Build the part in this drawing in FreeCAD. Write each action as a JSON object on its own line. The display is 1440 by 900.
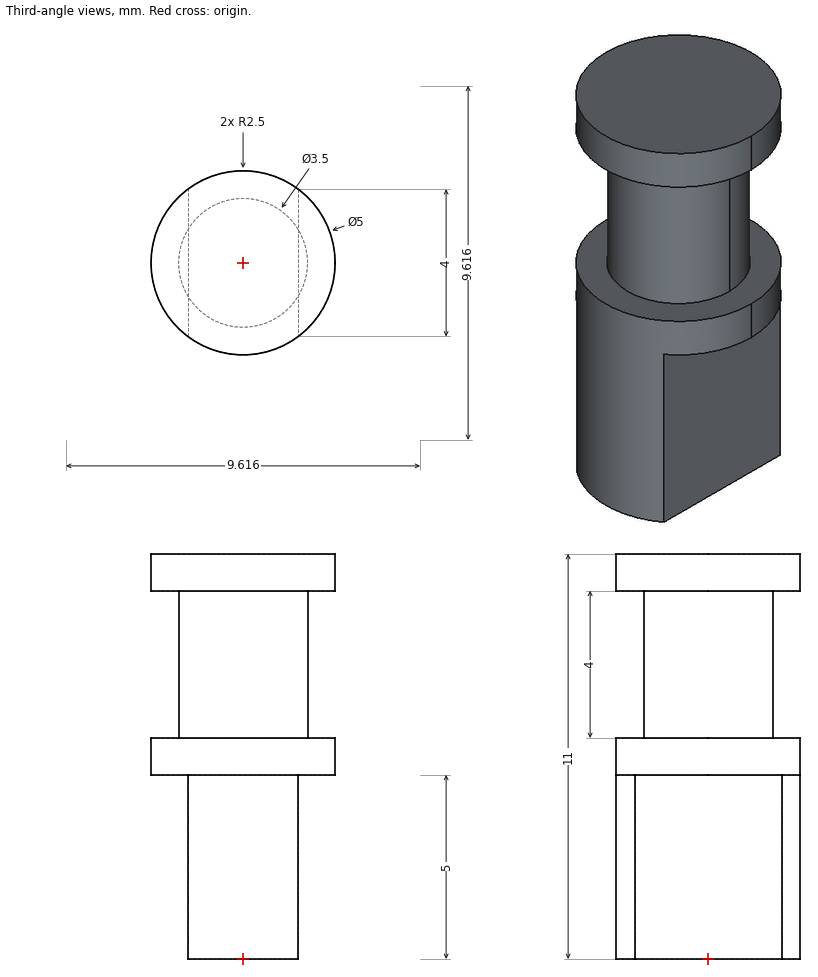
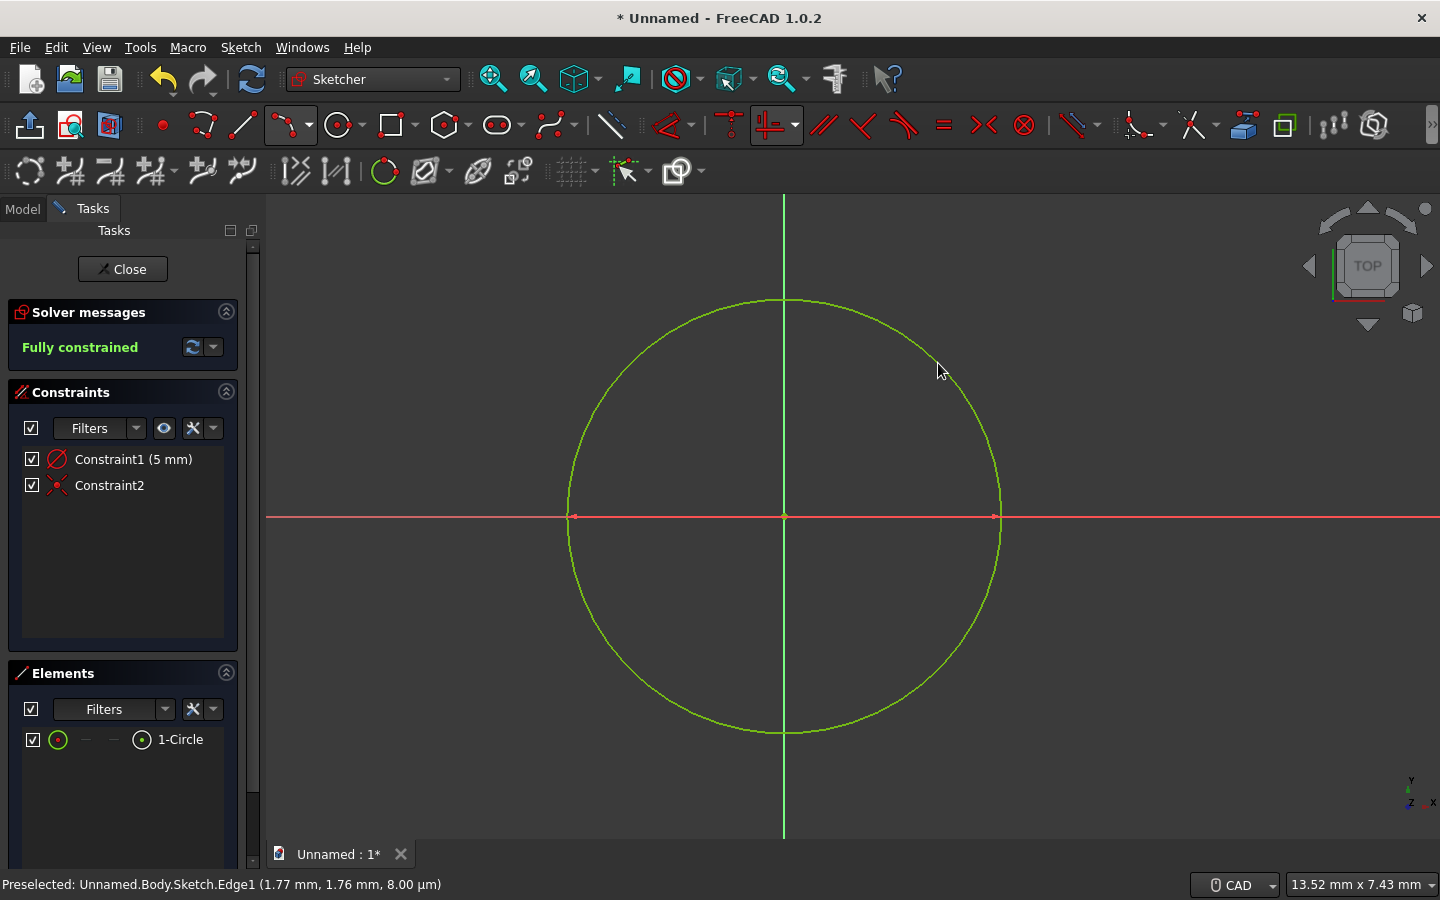
{"action": "left_click", "coordinate": [123, 269]}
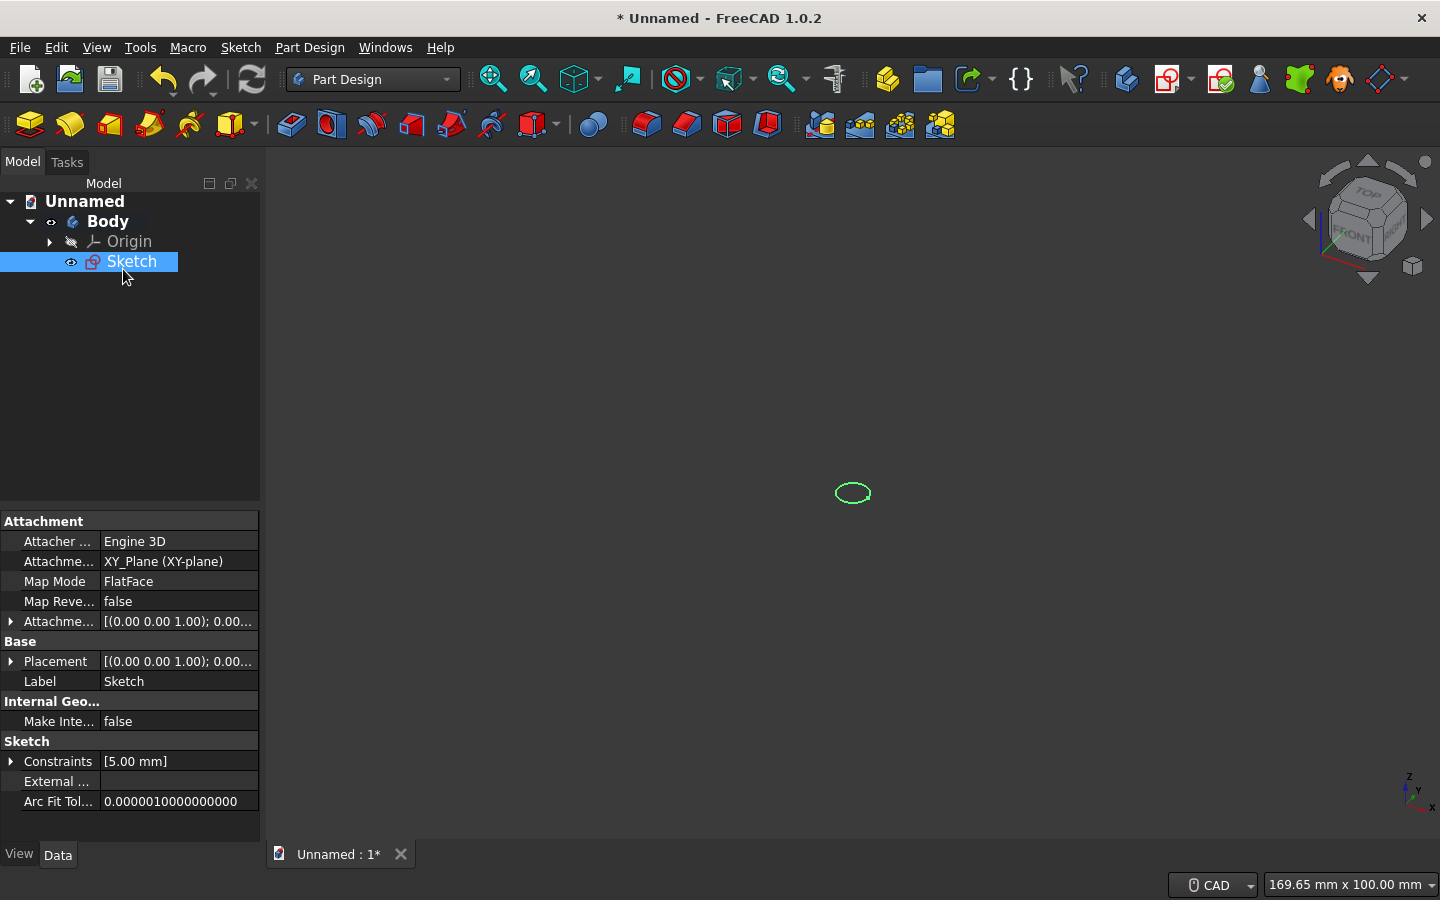
{"action": "left_click", "coordinate": [30, 124]}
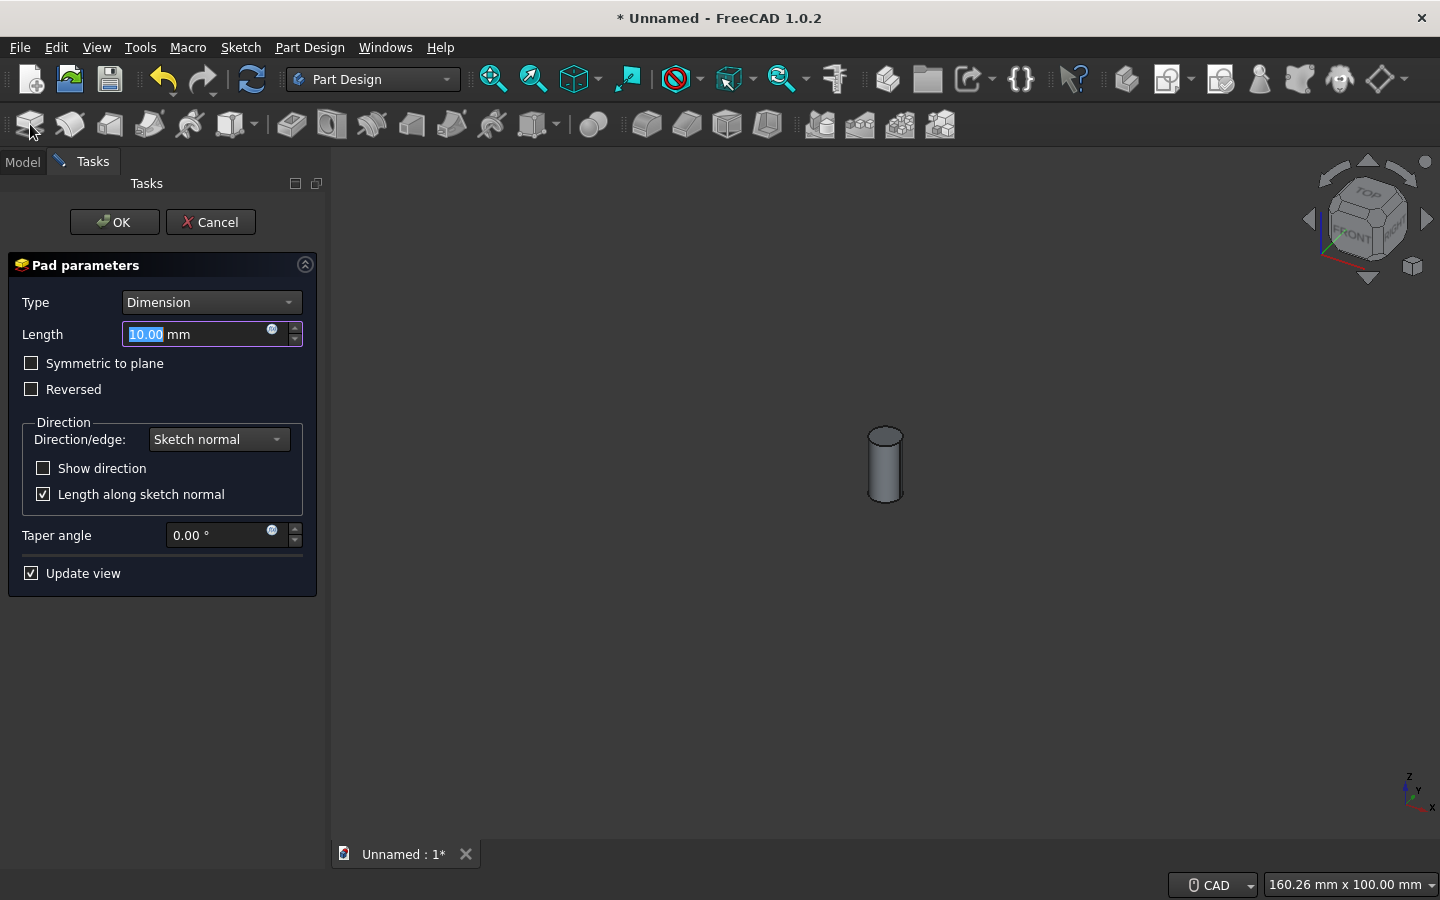
{"action": "type", "text": "11"}
{"action": "key", "text": "Tab"}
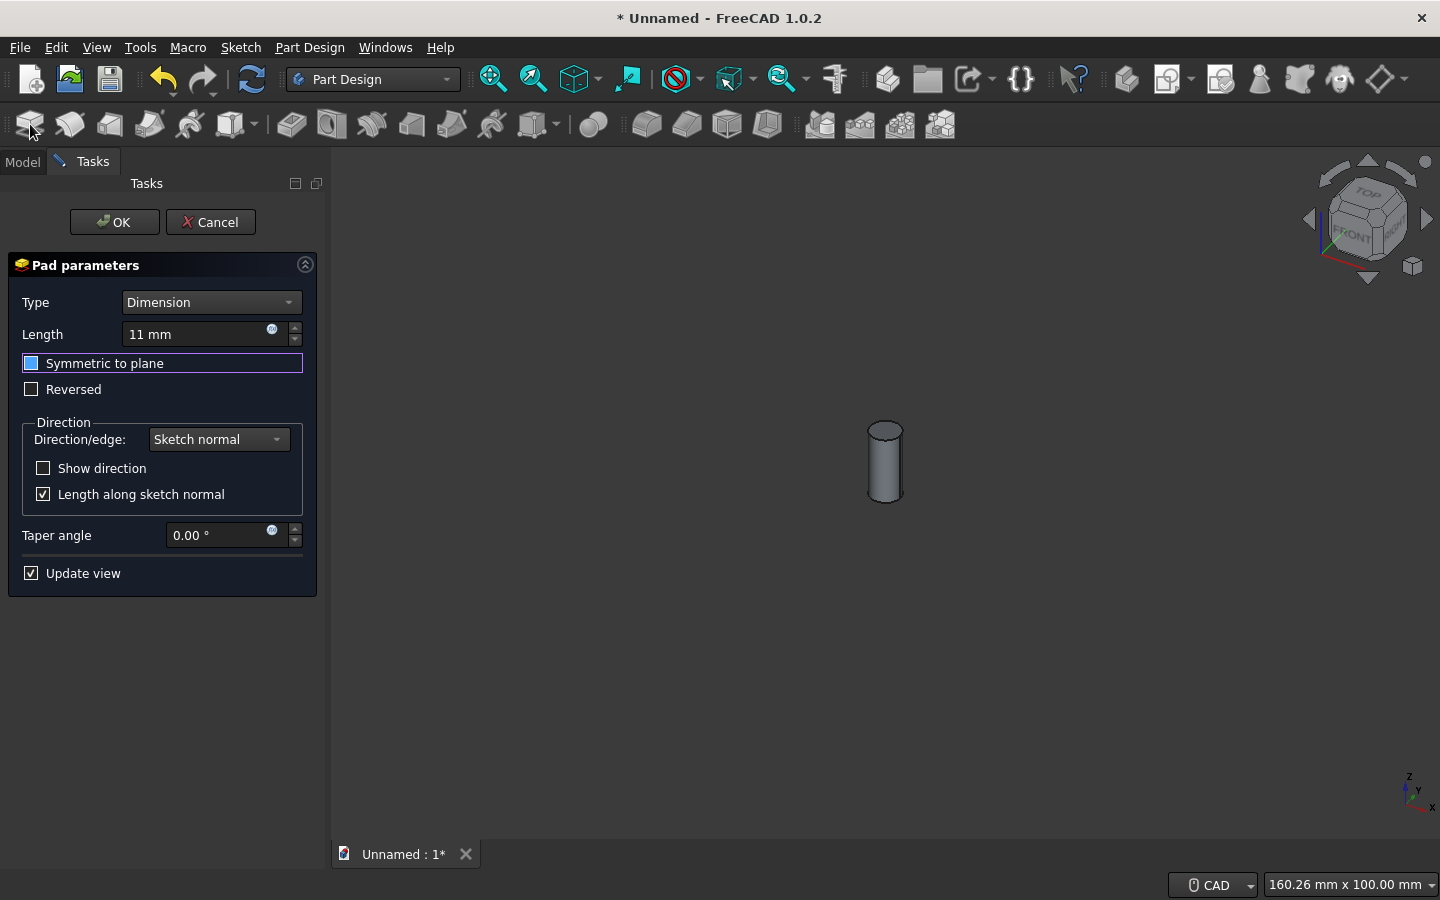
{"action": "left_click", "coordinate": [115, 222]}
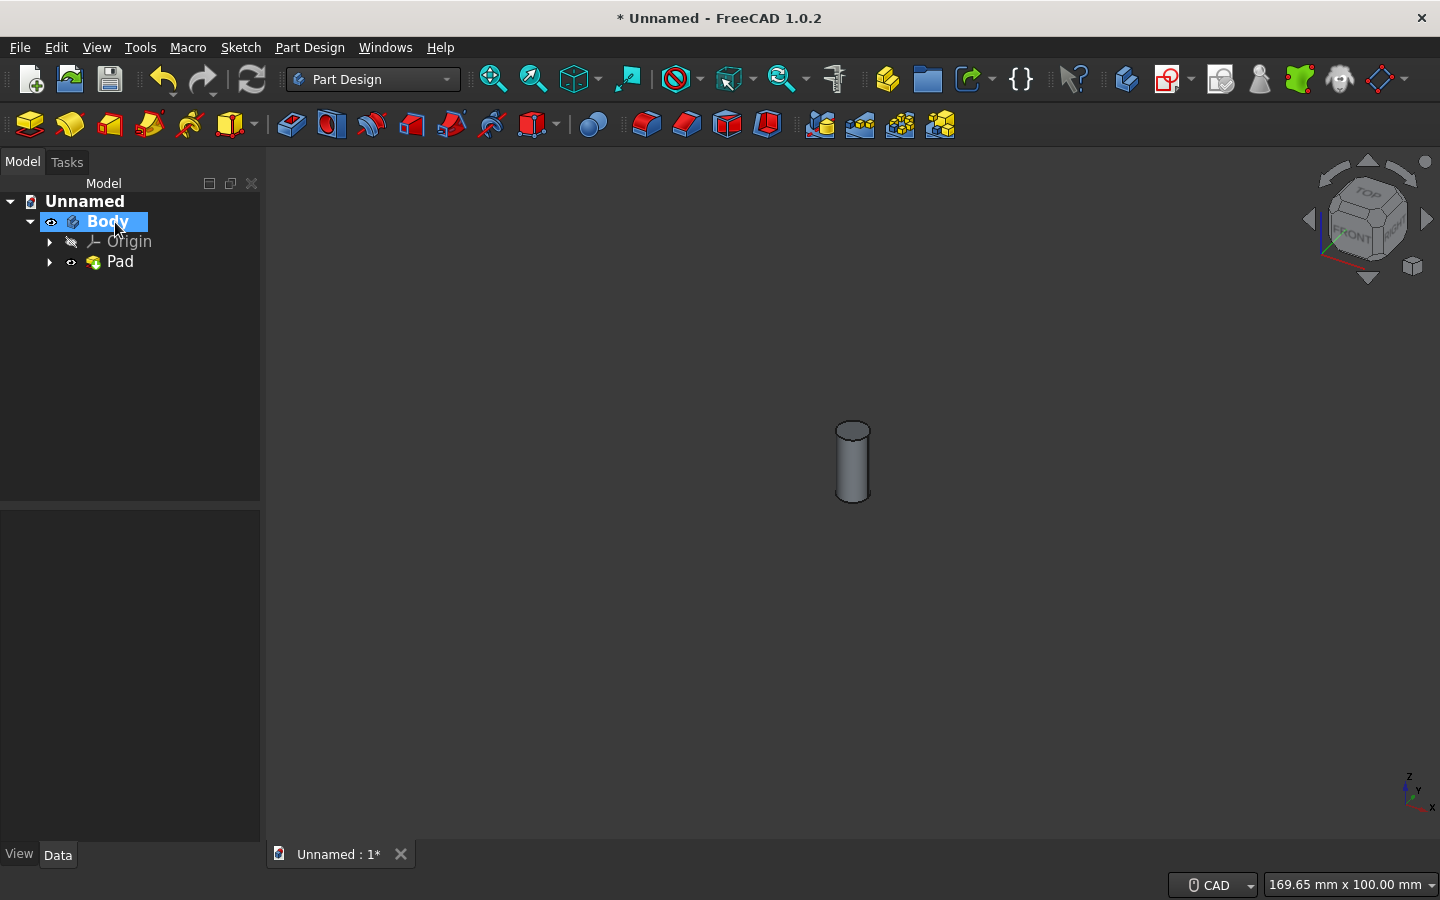
{"action": "left_click", "coordinate": [494, 80]}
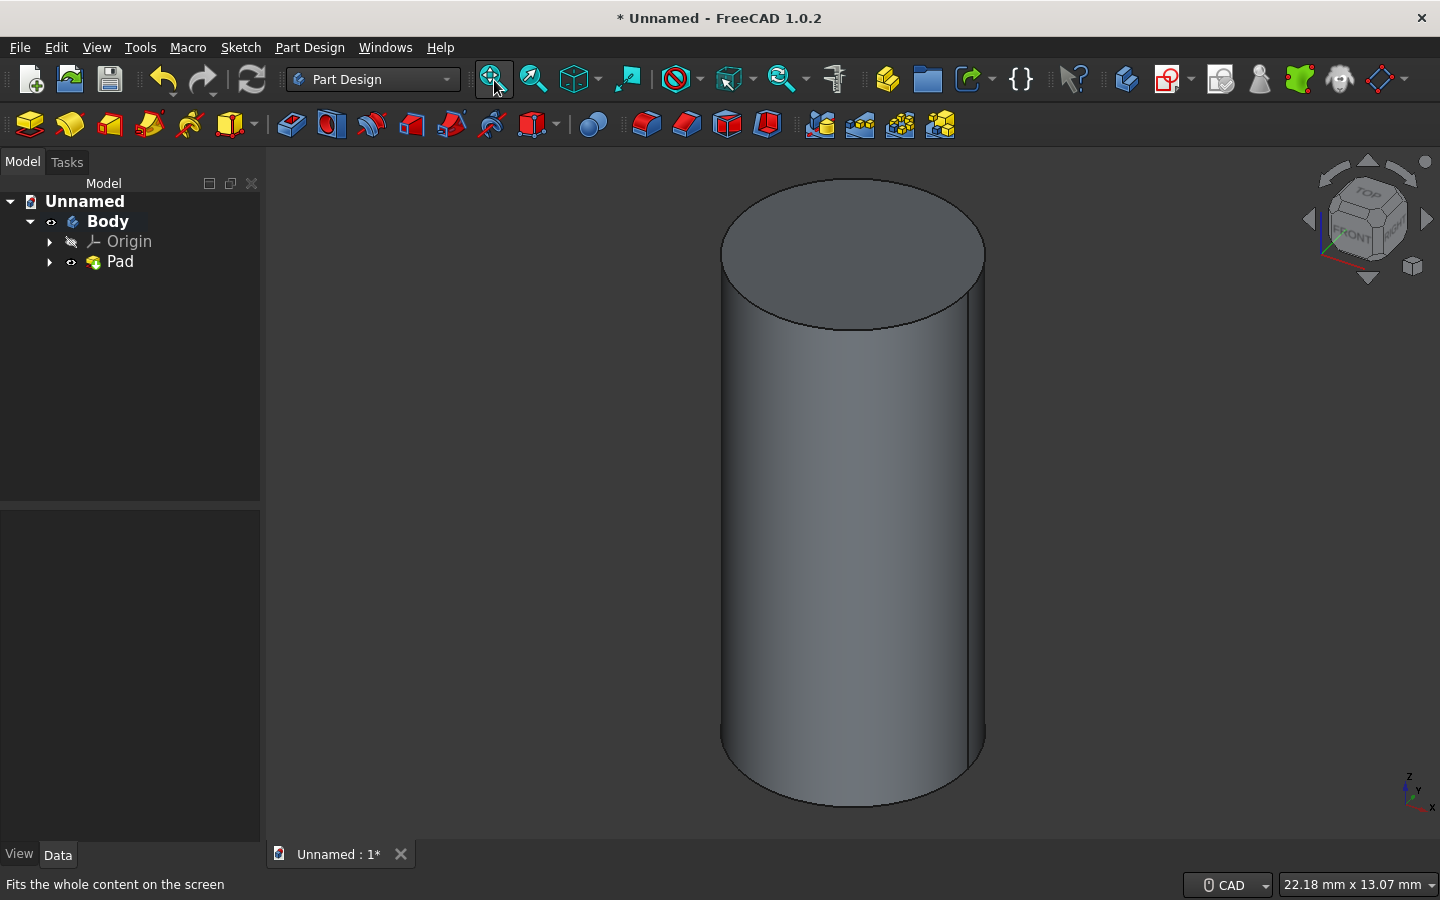
{"action": "left_click", "coordinate": [1168, 80]}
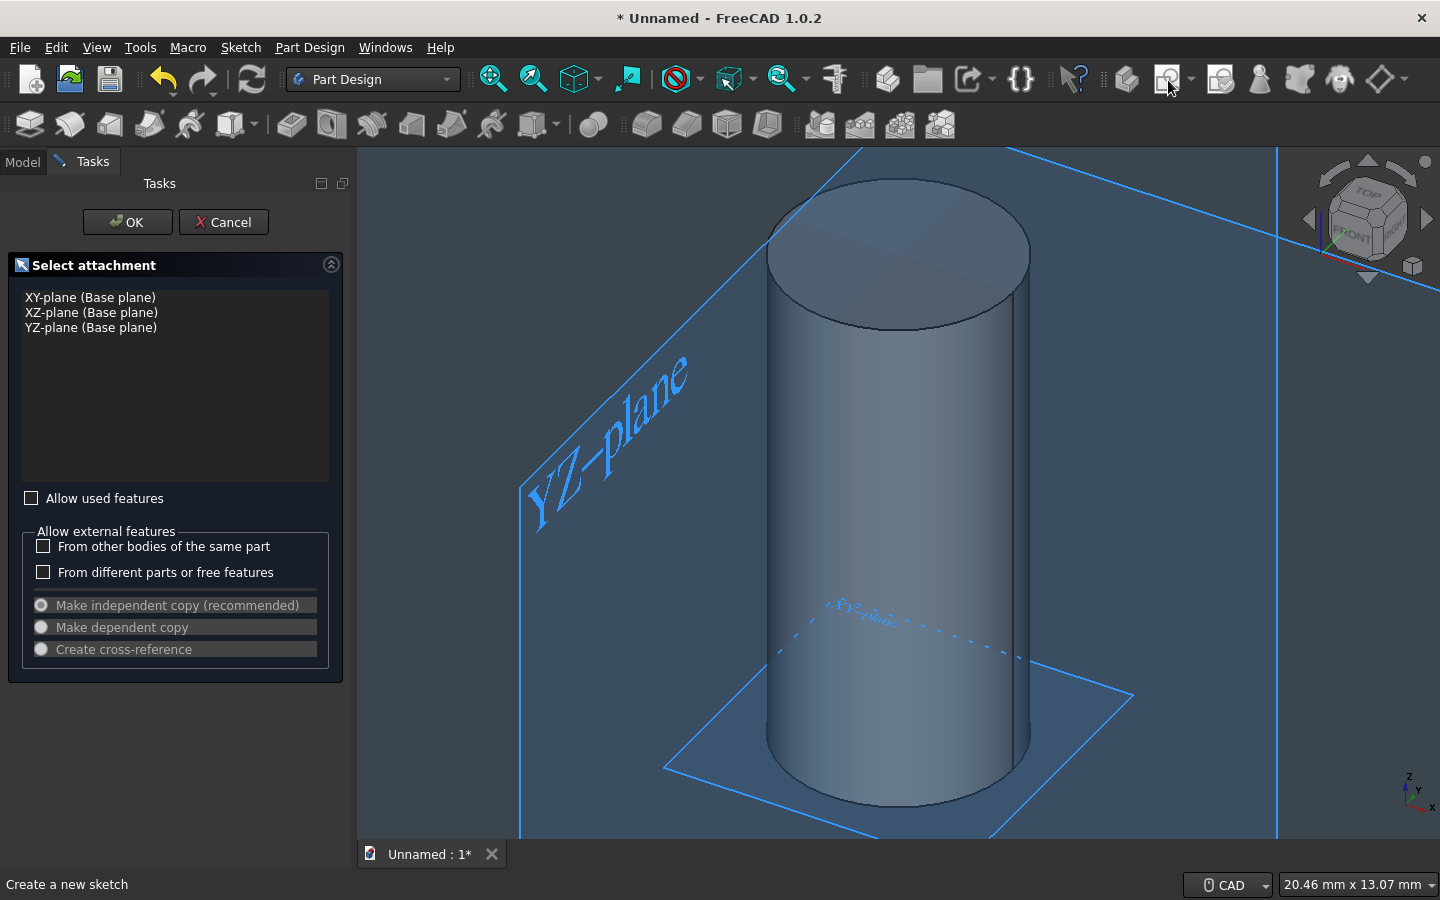
{"action": "left_click", "coordinate": [82, 298]}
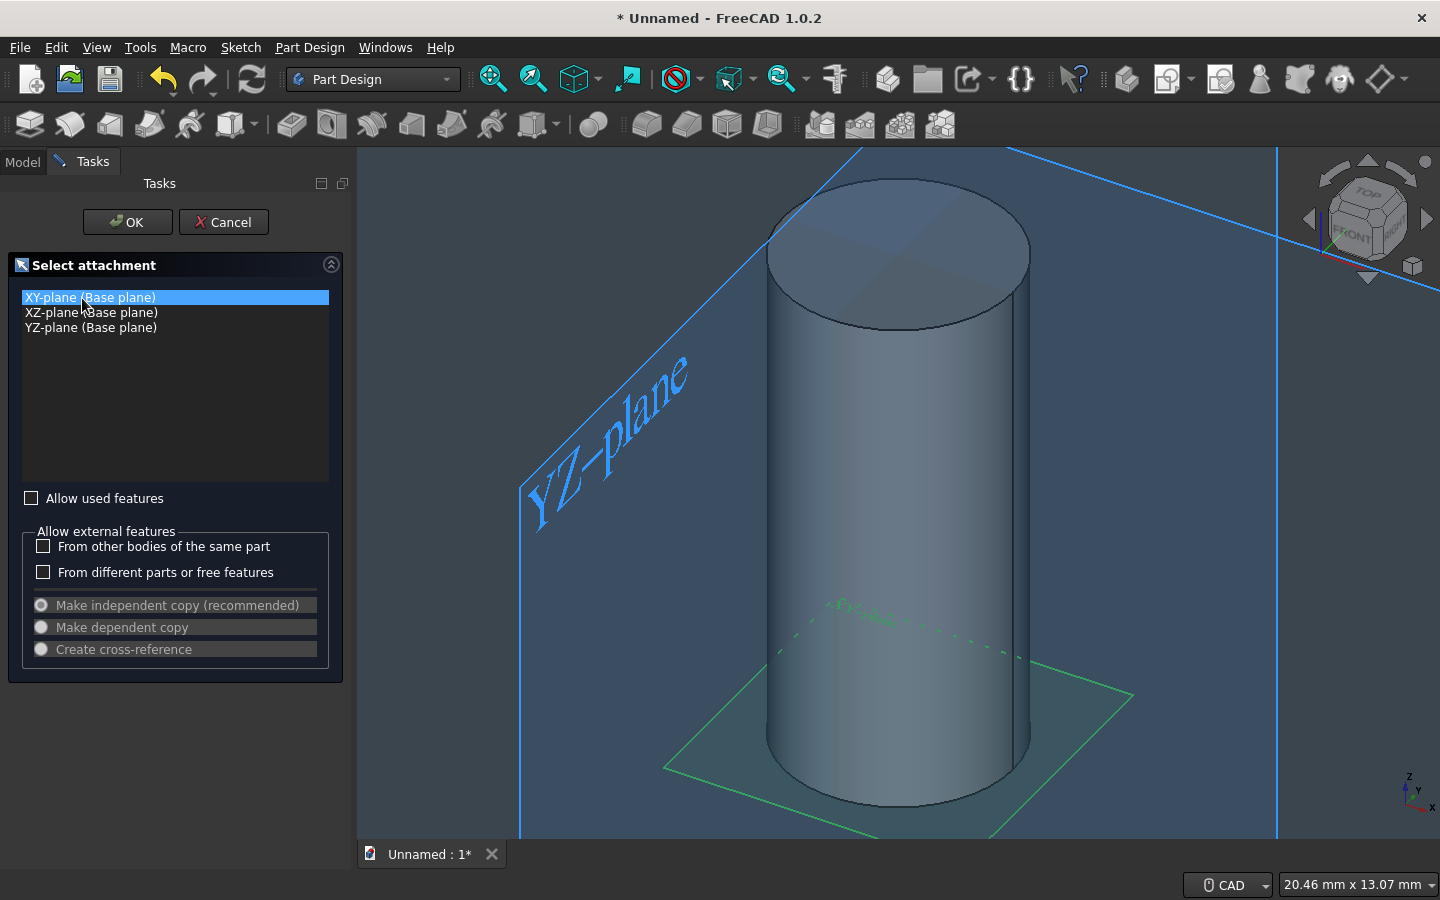
{"action": "left_click", "coordinate": [128, 222]}